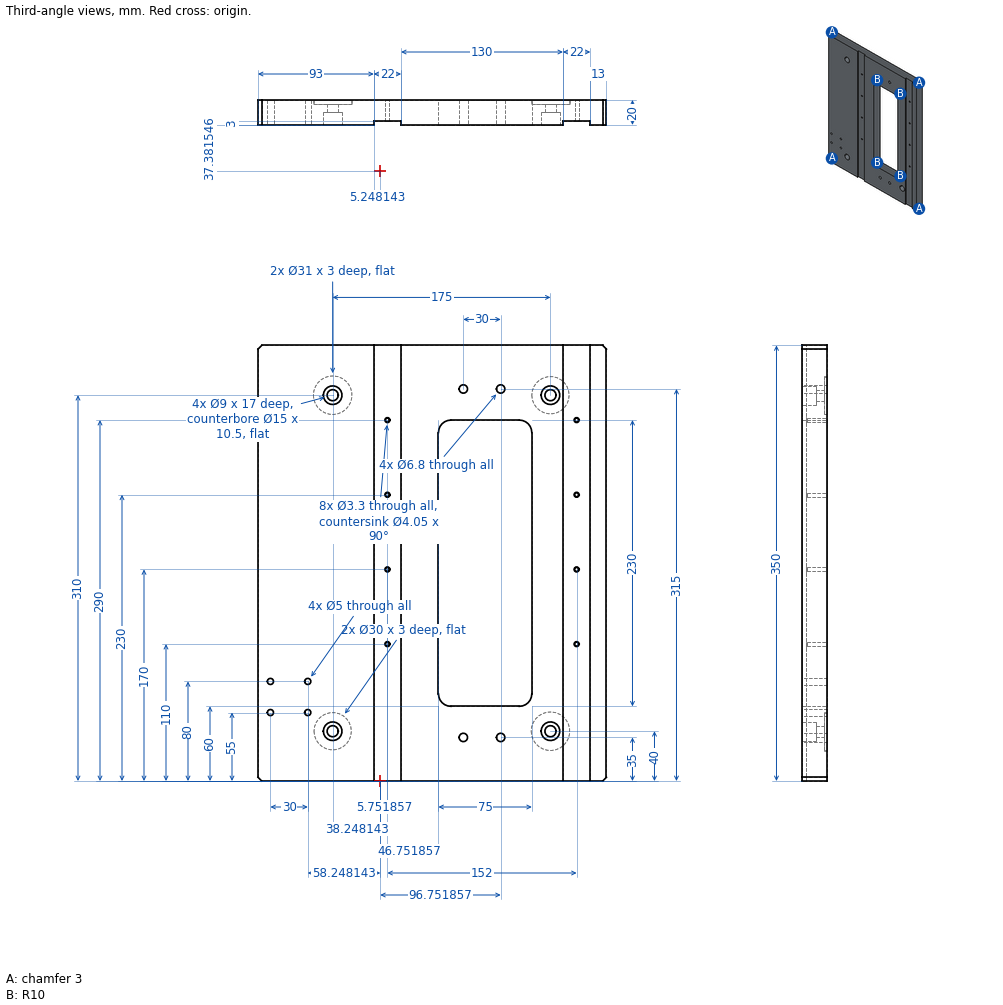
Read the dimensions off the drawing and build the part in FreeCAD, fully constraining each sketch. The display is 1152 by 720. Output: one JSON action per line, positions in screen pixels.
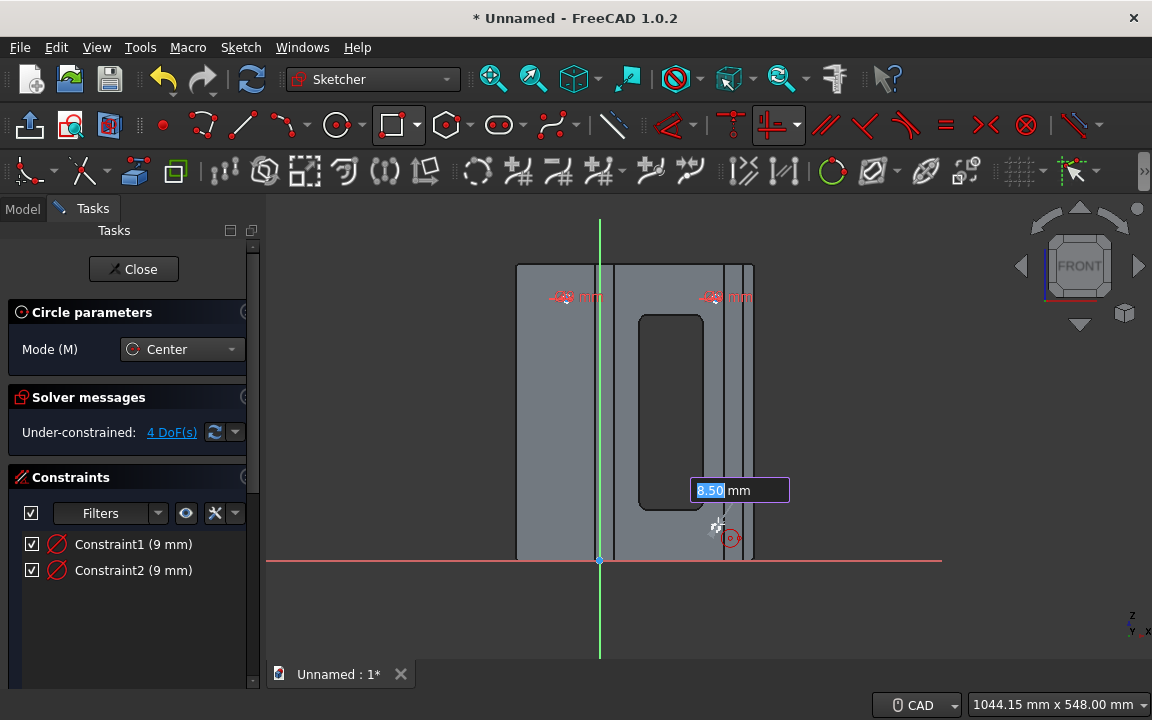
{"action": "type", "text": "9"}
{"action": "key", "text": "Return"}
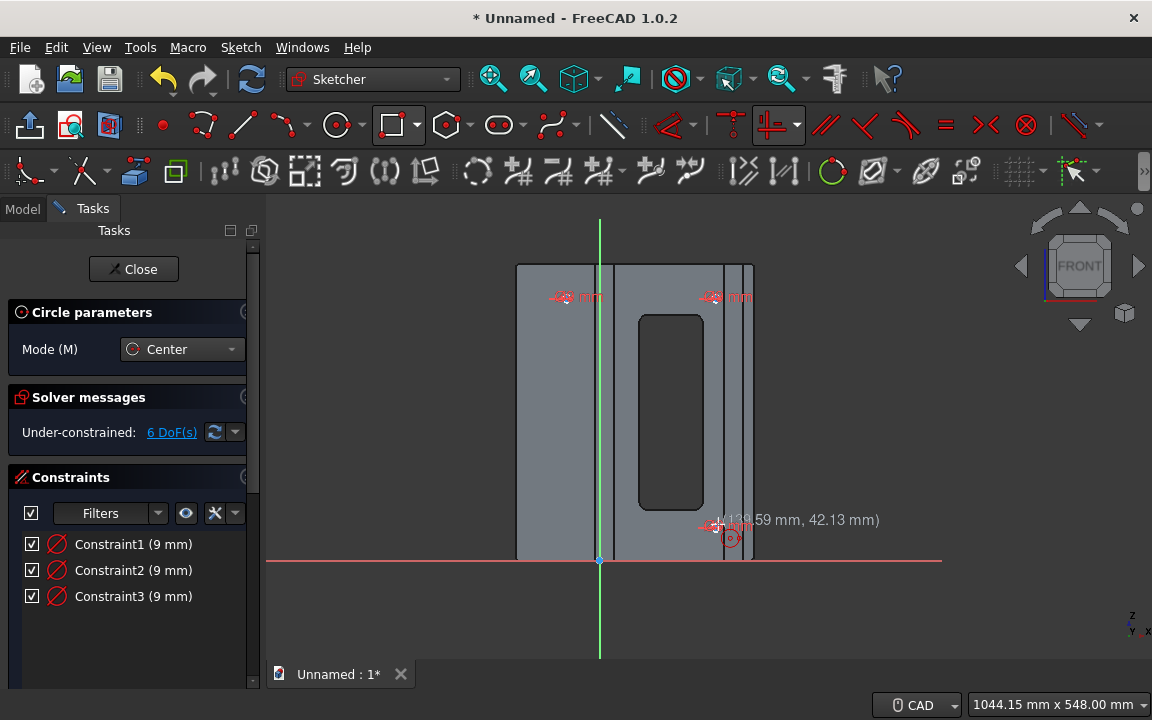
{"action": "scroll", "coordinate": [567, 527], "scroll_direction": "up", "scroll_amount": 9}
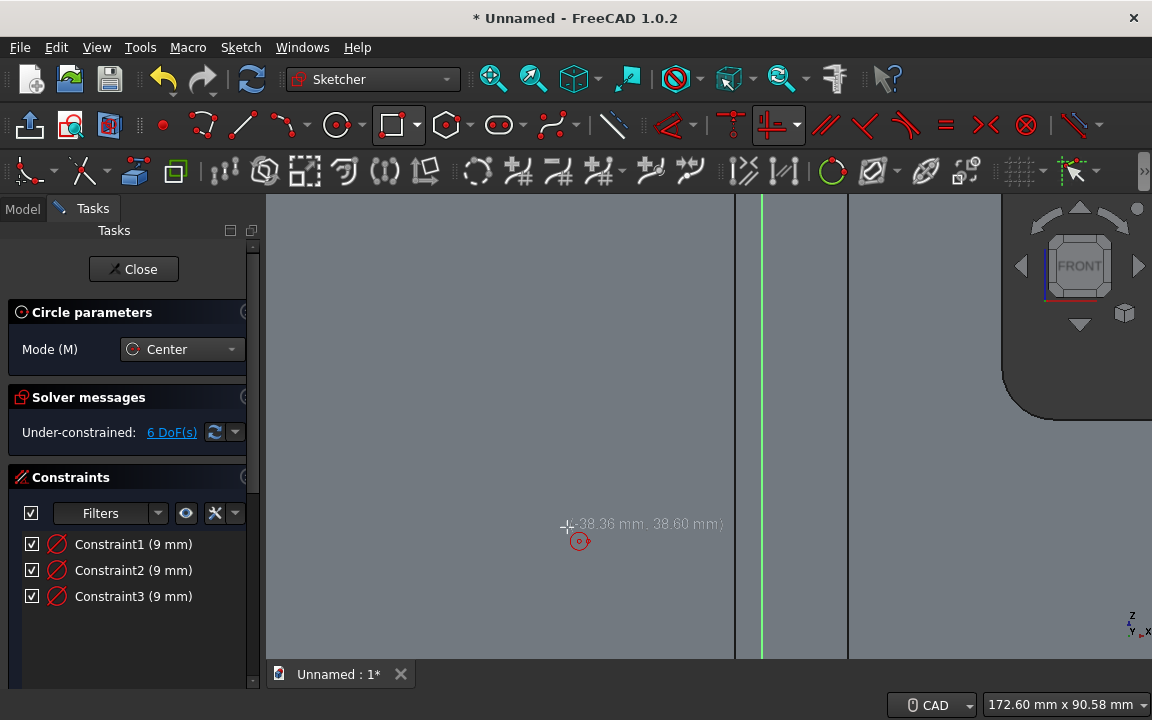
{"action": "scroll", "coordinate": [566, 527], "scroll_direction": "down", "scroll_amount": 9}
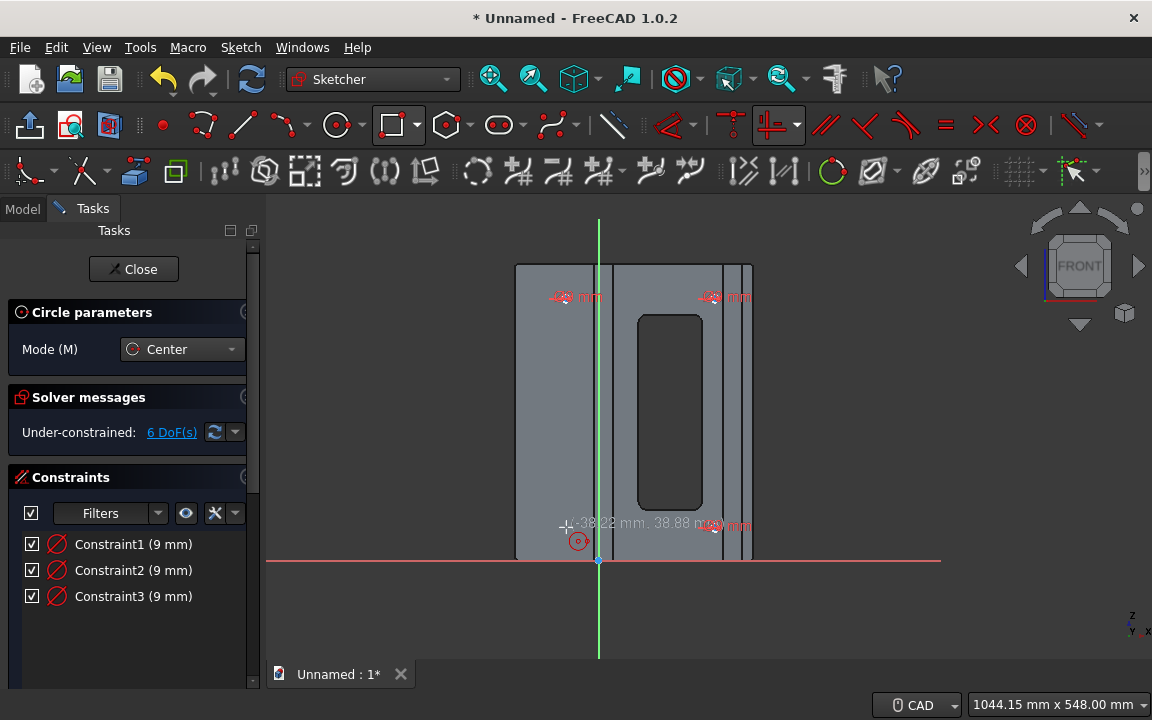
{"action": "left_click", "coordinate": [566, 527]}
{"action": "mouse_move", "coordinate": [569, 524]}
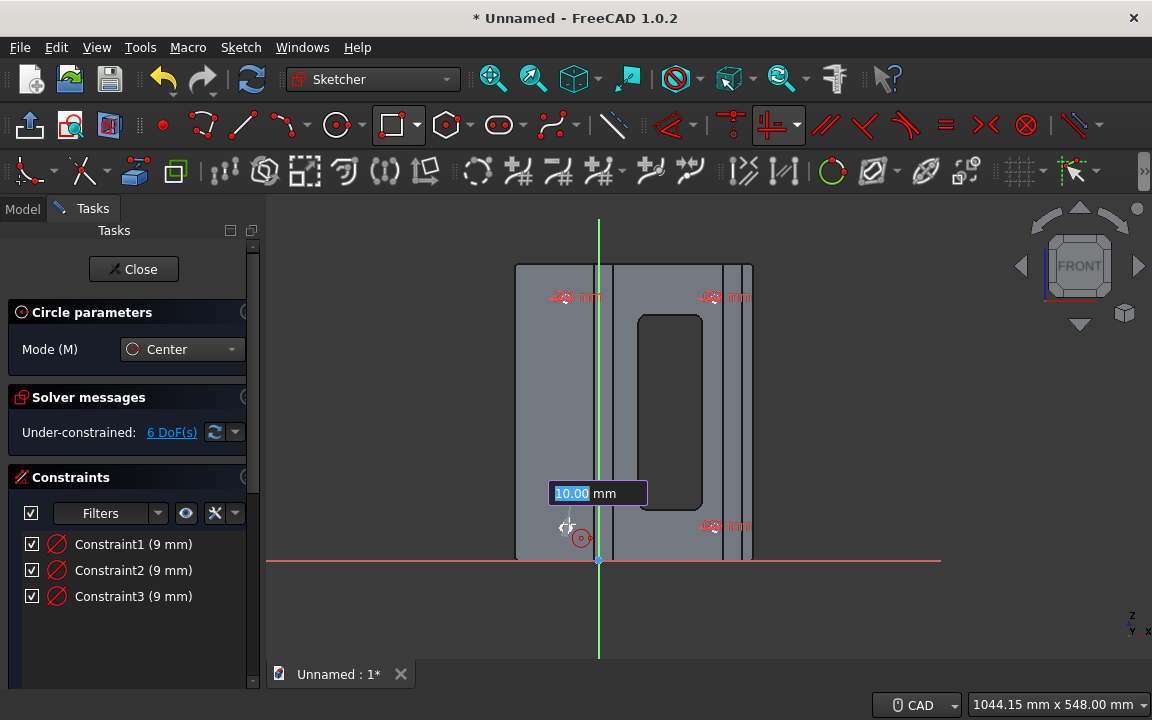
{"action": "type", "text": "9"}
{"action": "key", "text": "Return"}
{"action": "key", "text": "Escape"}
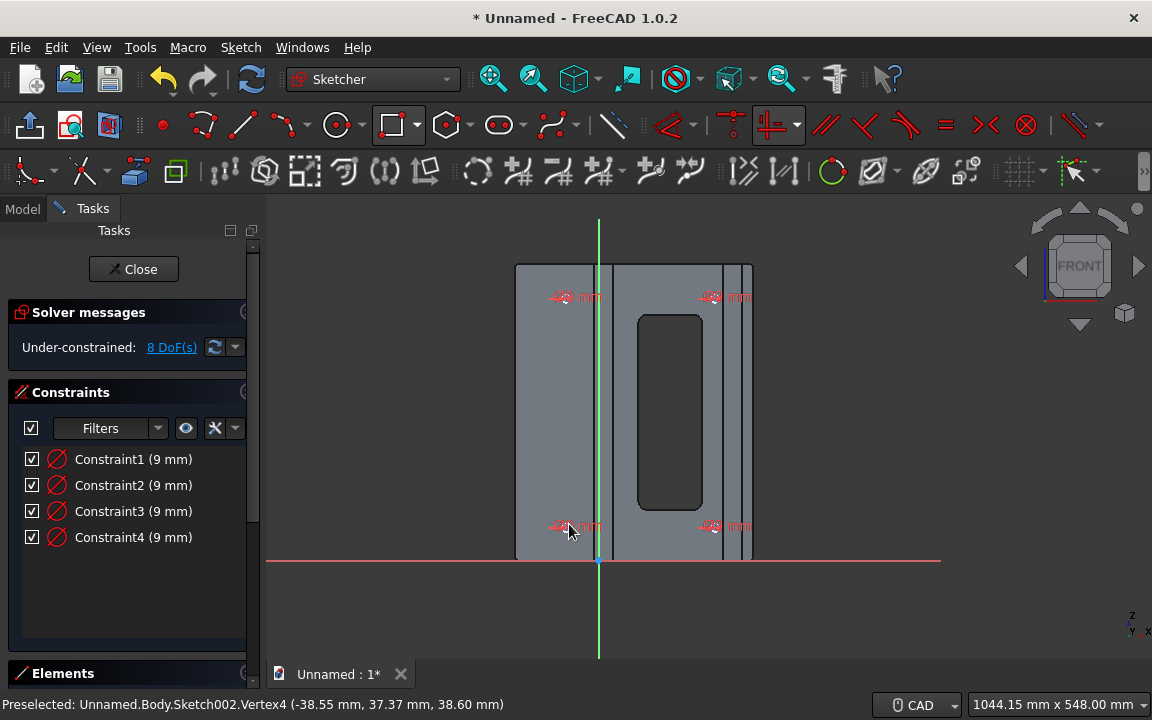
{"action": "left_click", "coordinate": [566, 299]}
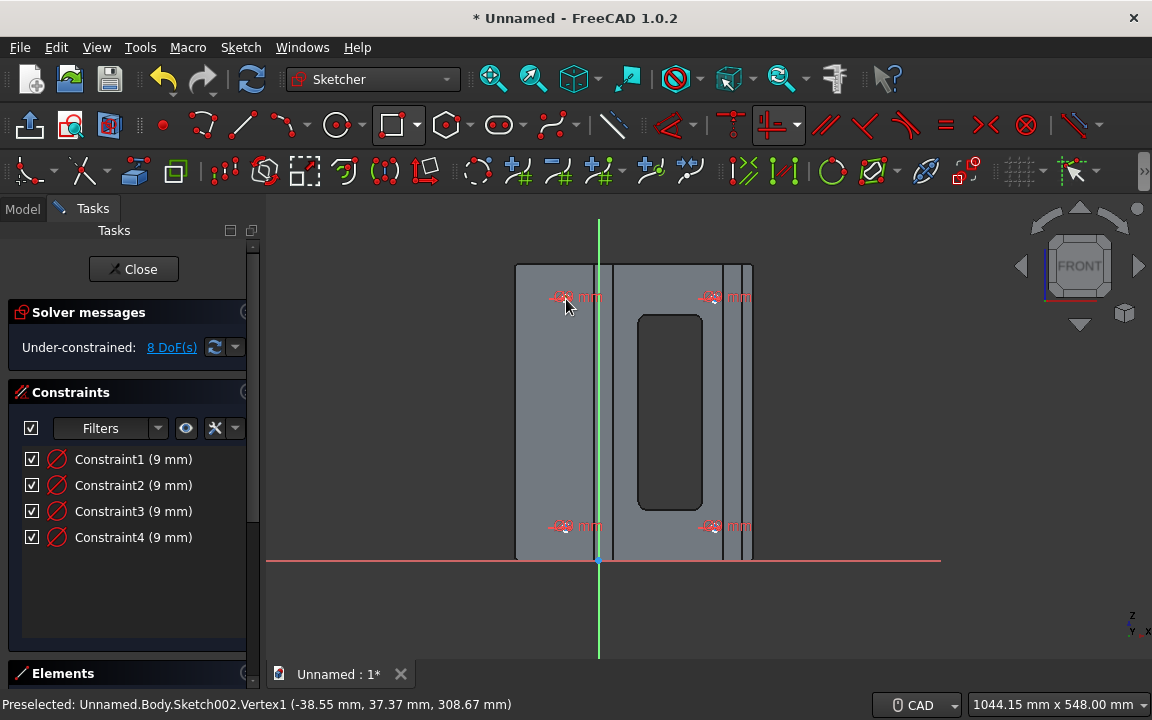
{"action": "left_click", "coordinate": [715, 299]}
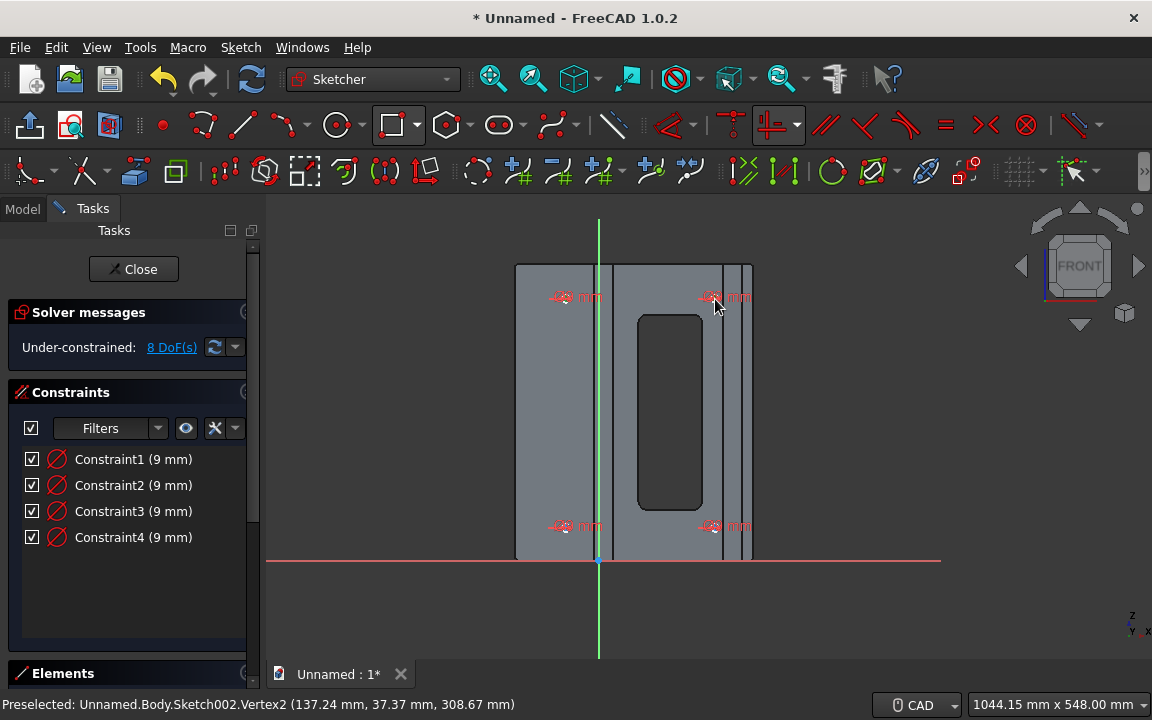
{"action": "key", "text": "h"}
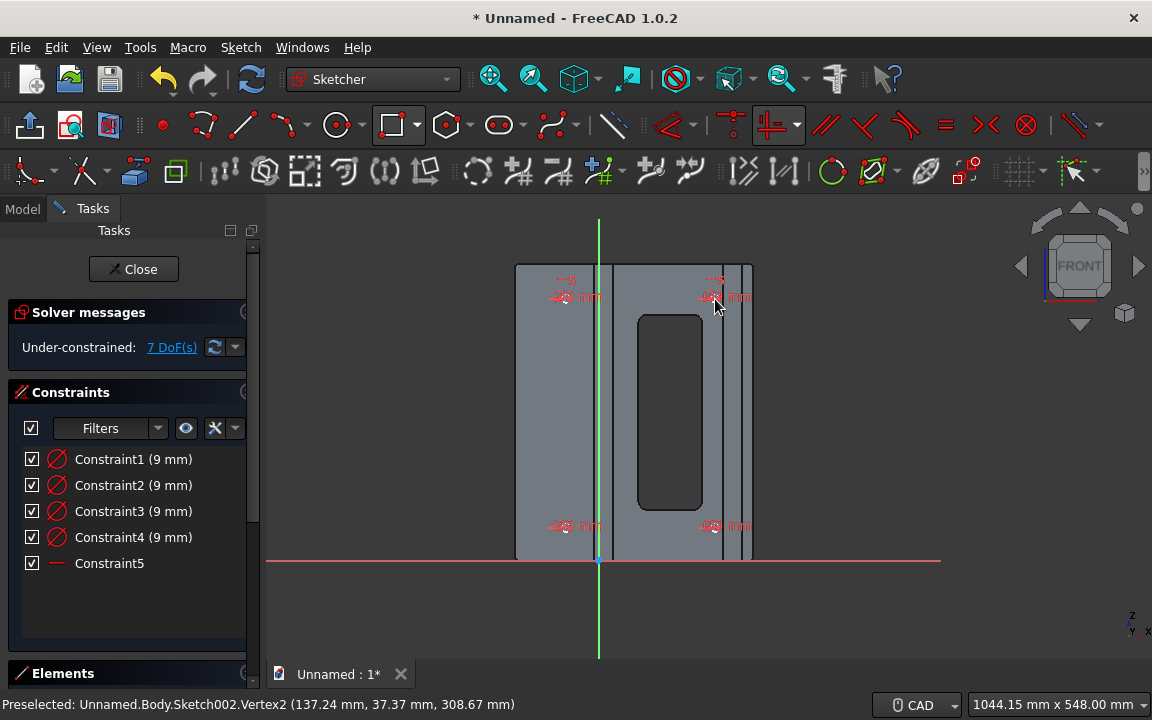
{"action": "left_click", "coordinate": [715, 299]}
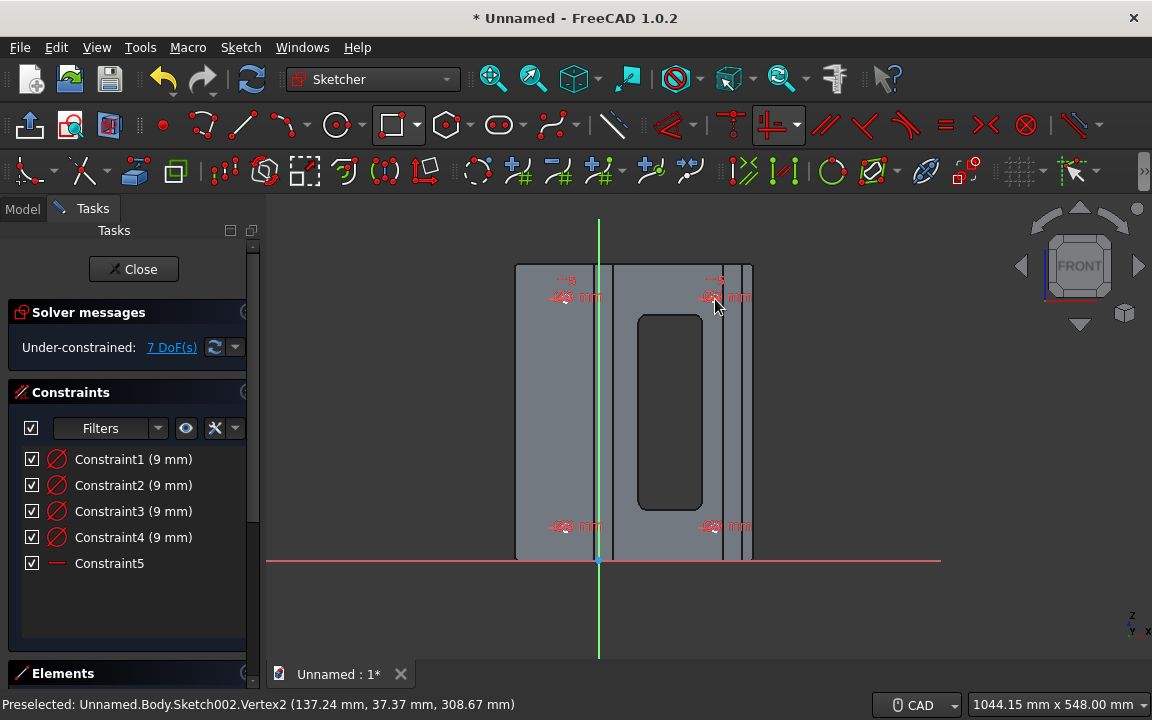
{"action": "left_click", "coordinate": [715, 528]}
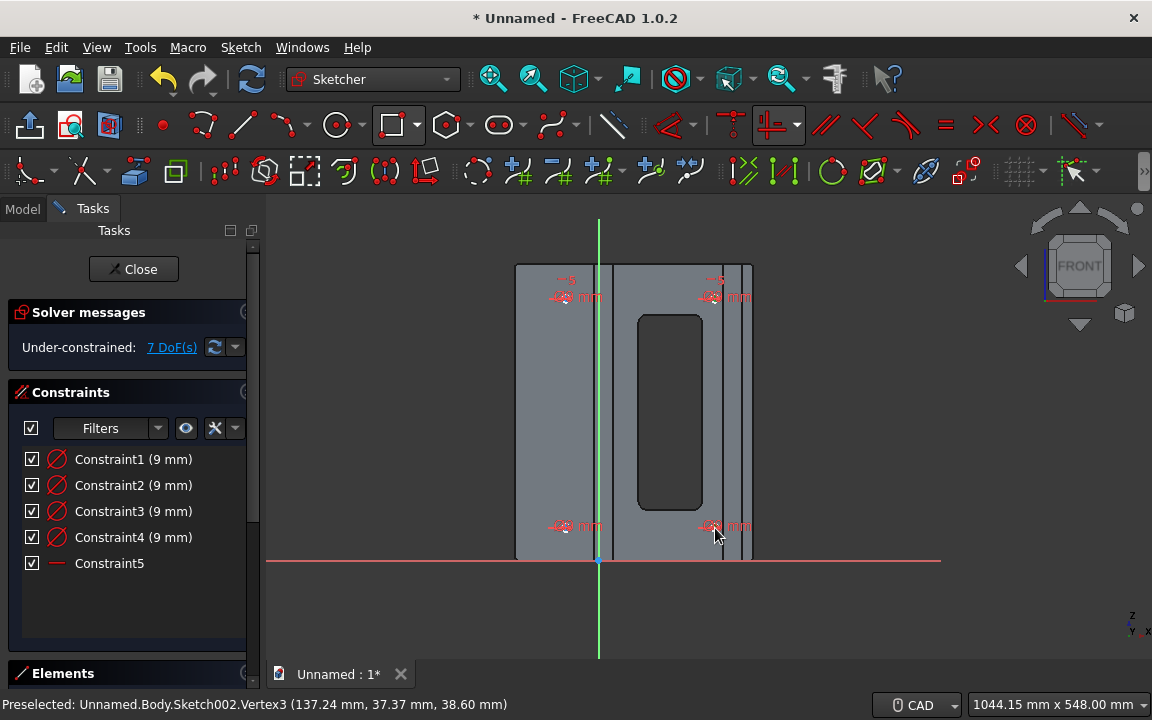
{"action": "key", "text": "v"}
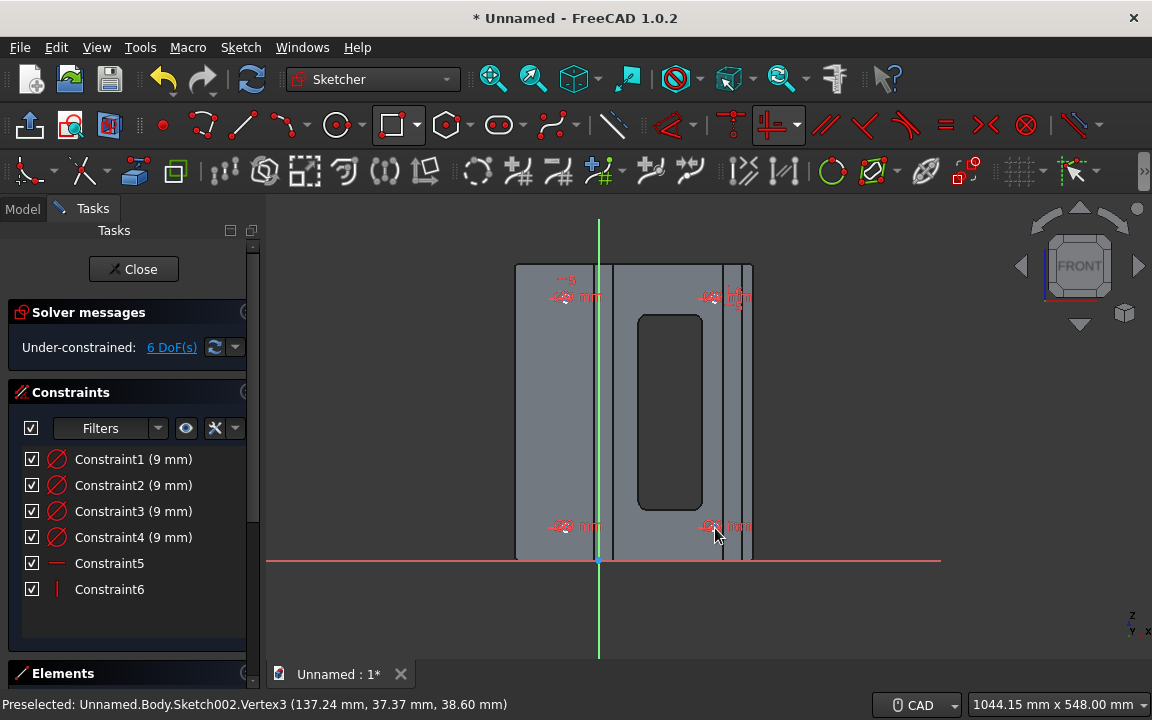
{"action": "left_click", "coordinate": [566, 299]}